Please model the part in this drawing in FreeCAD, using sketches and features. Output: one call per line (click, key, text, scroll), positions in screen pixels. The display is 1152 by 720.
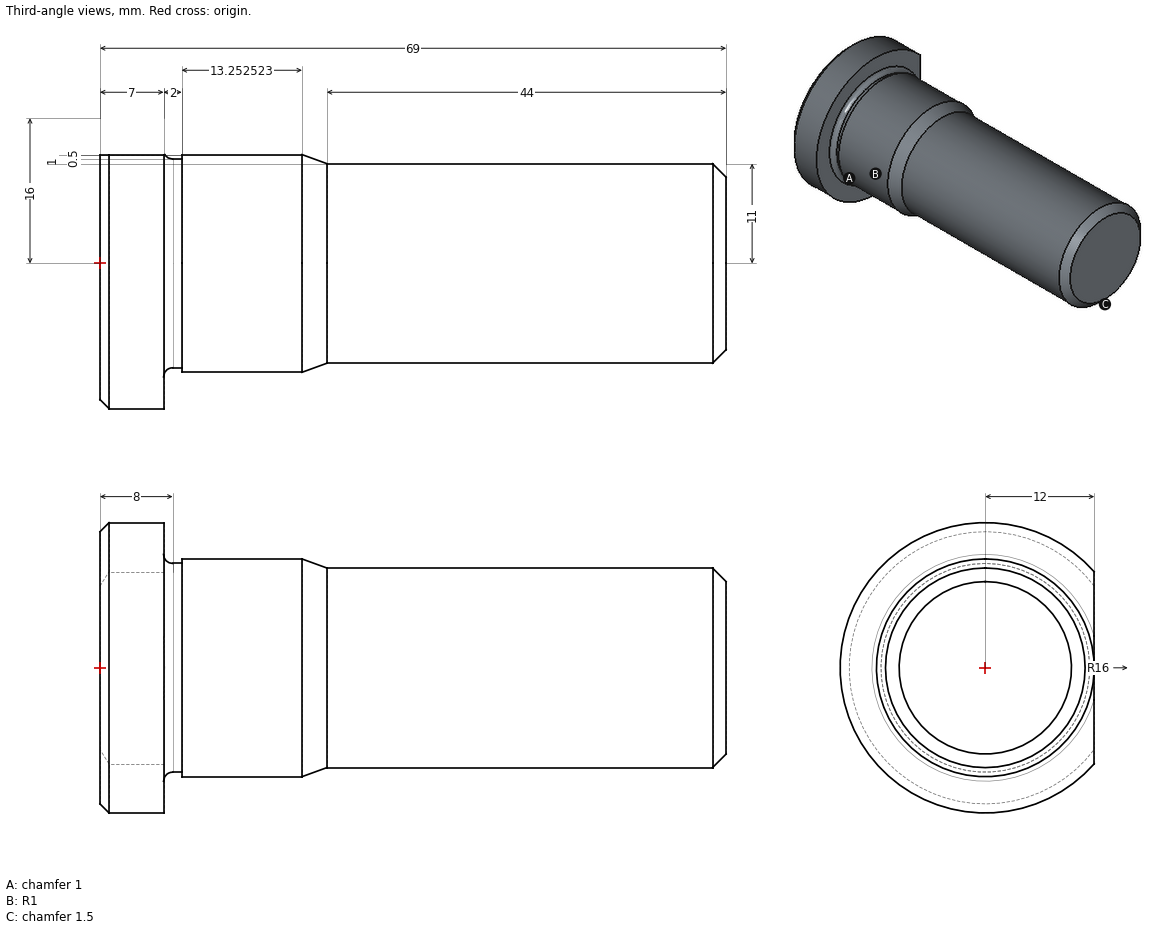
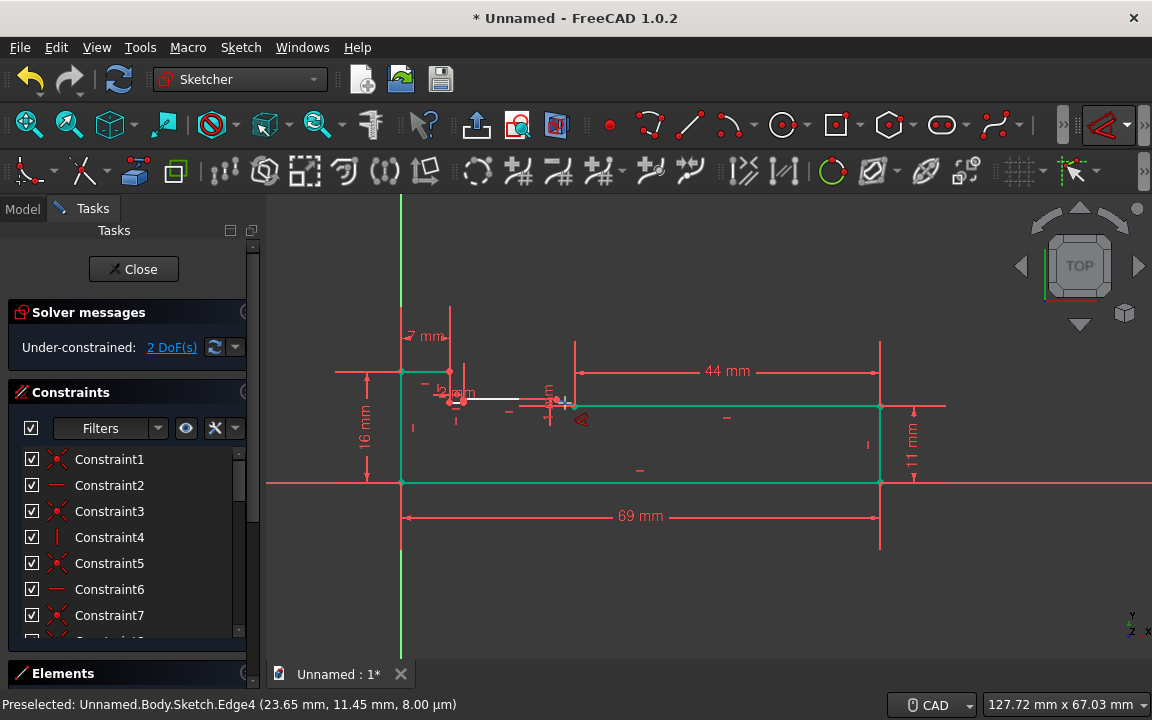
scroll(464, 401, up, 13)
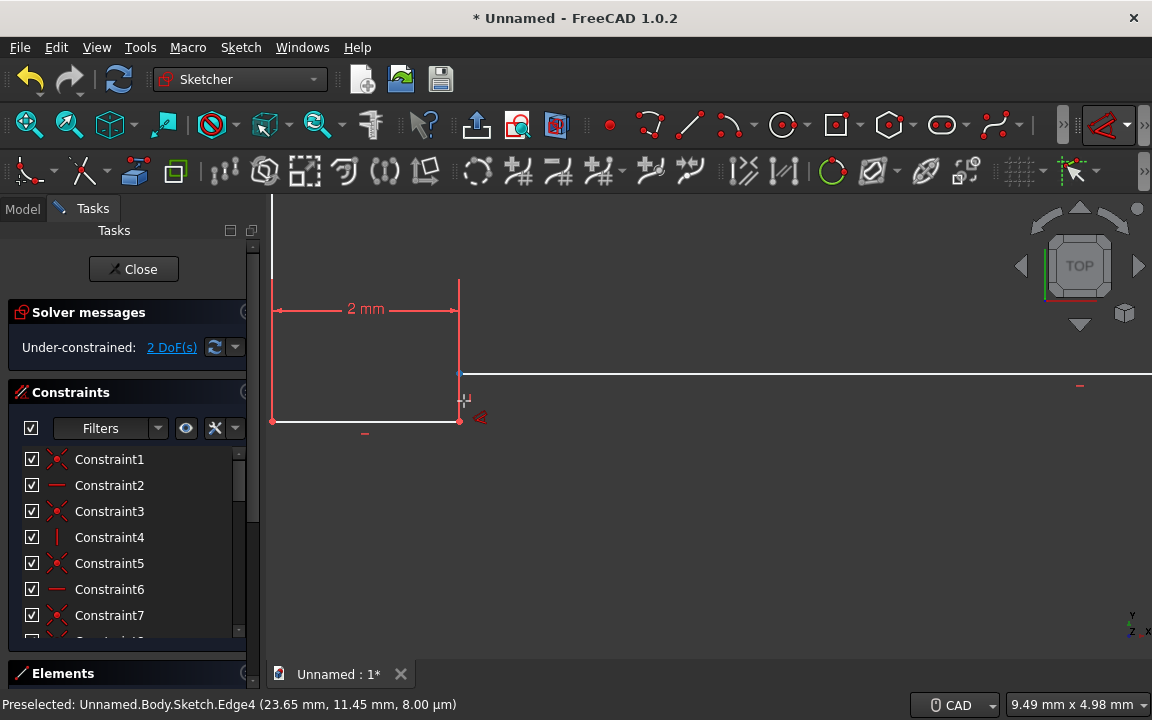
click(459, 398)
click(425, 398)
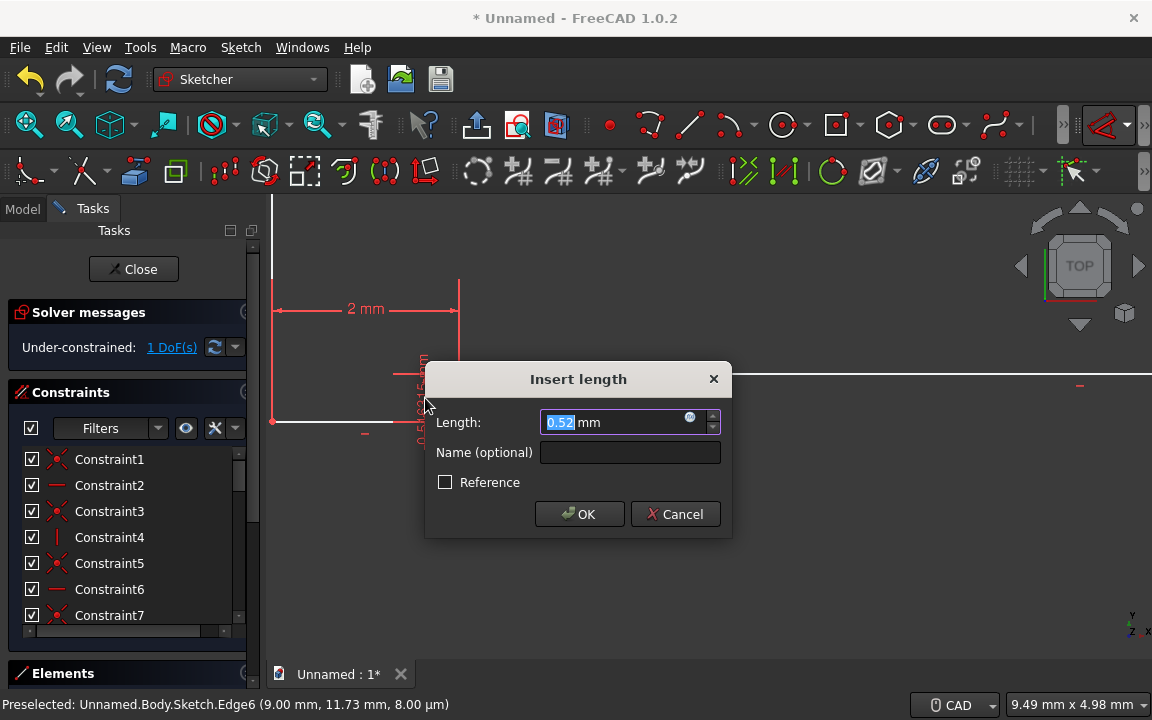
text(0.5)
key(Return)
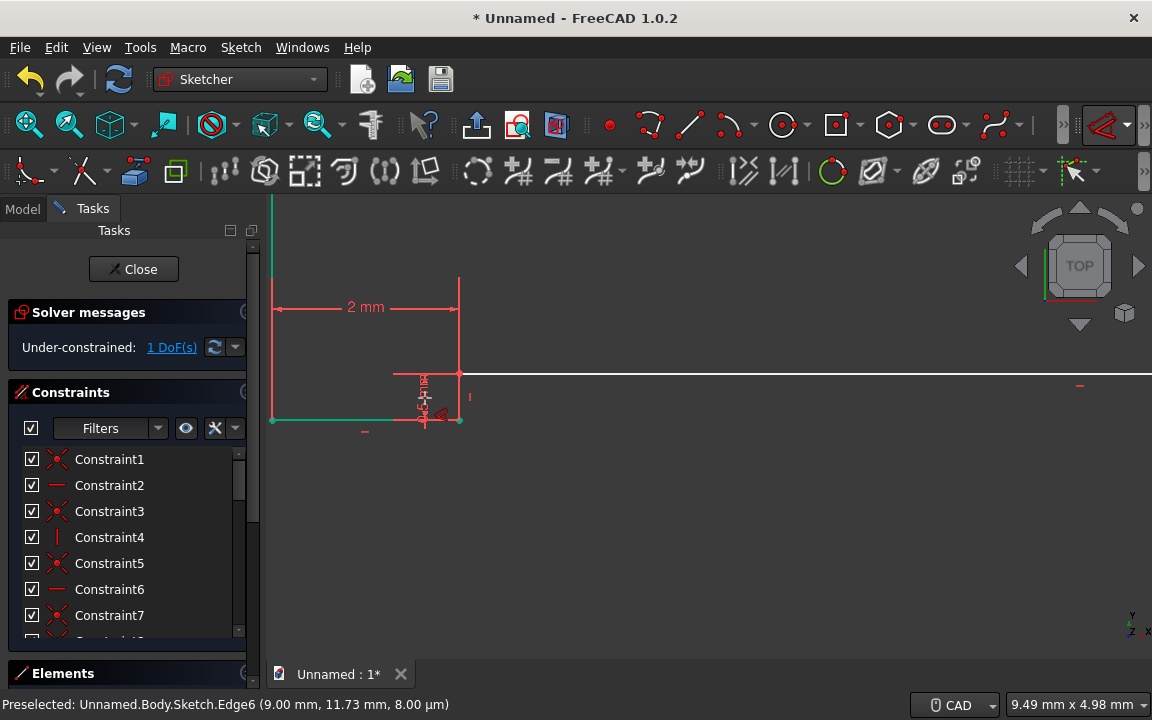
scroll(464, 401, down, 13)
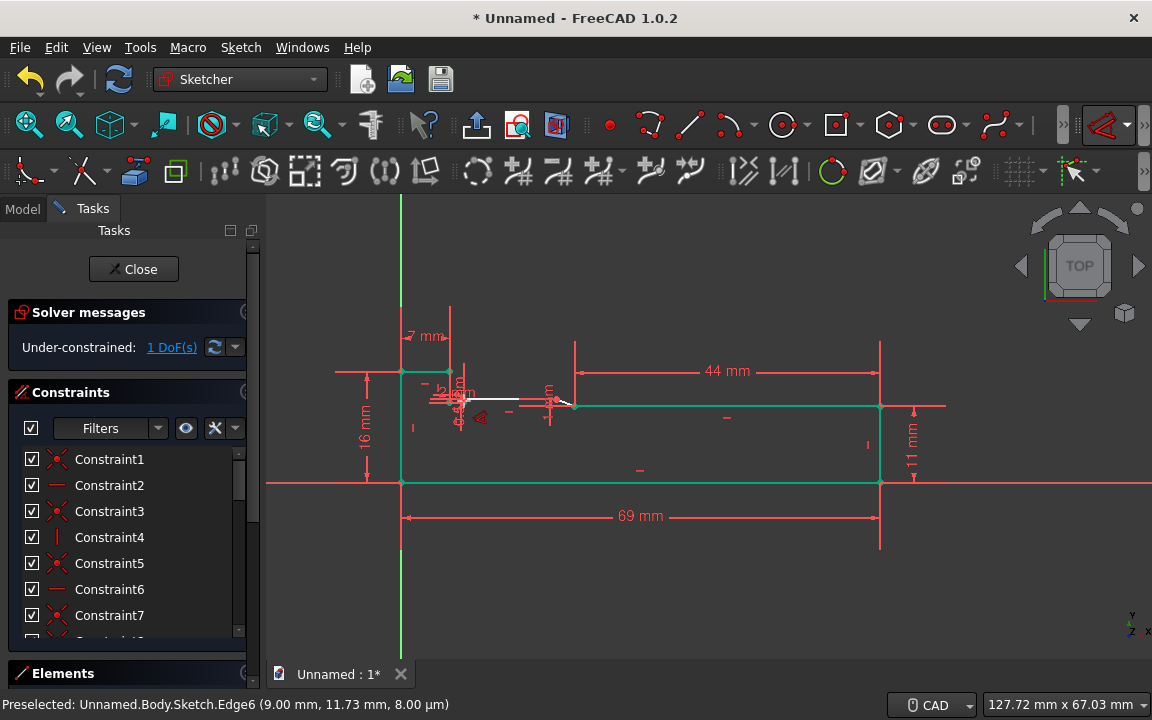
click(492, 399)
click(510, 365)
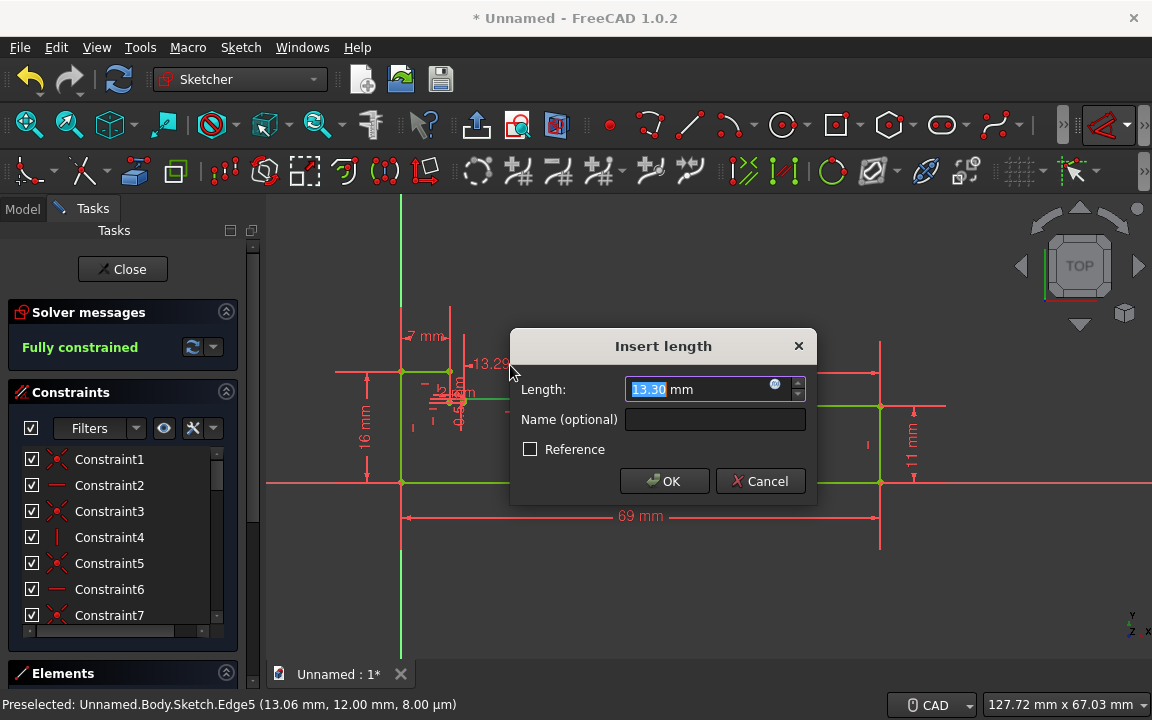
text(13.252523)
key(Return)
key(Escape)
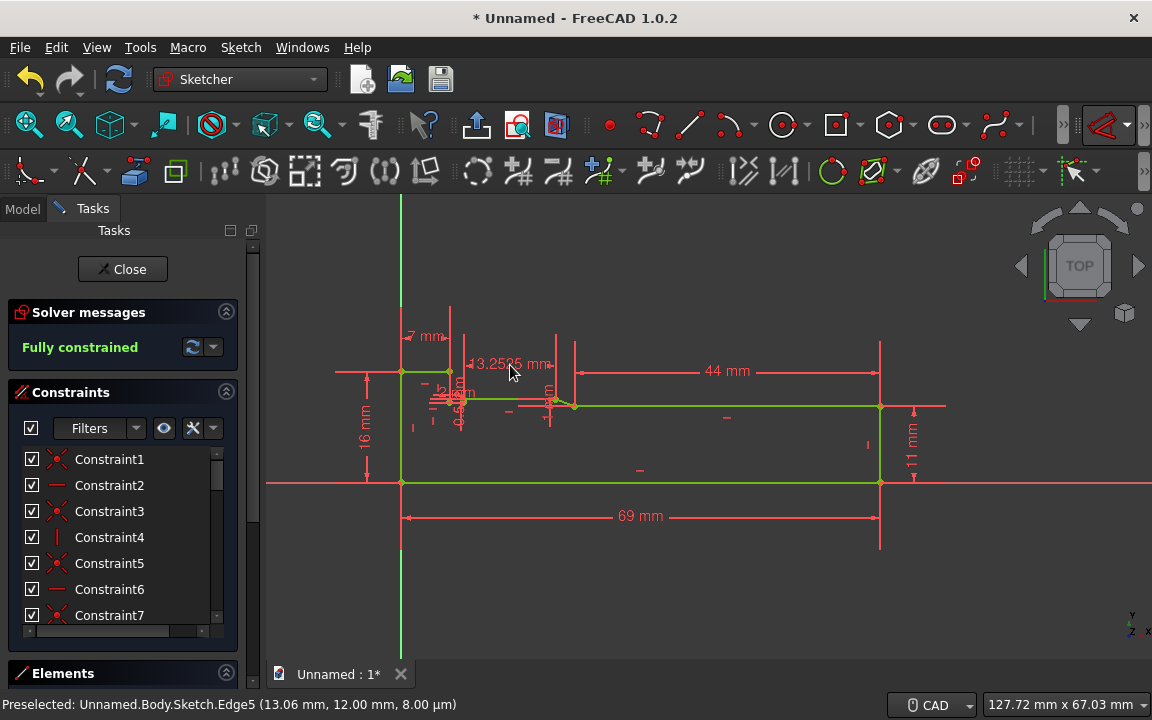
click(123, 269)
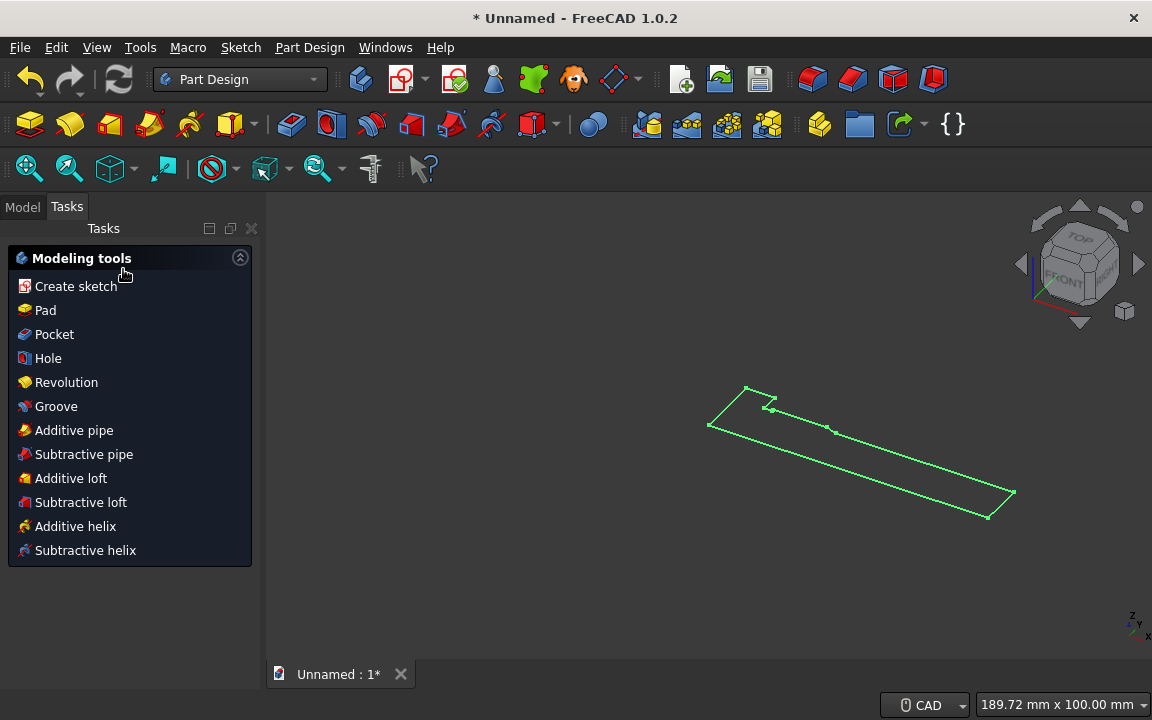
click(70, 124)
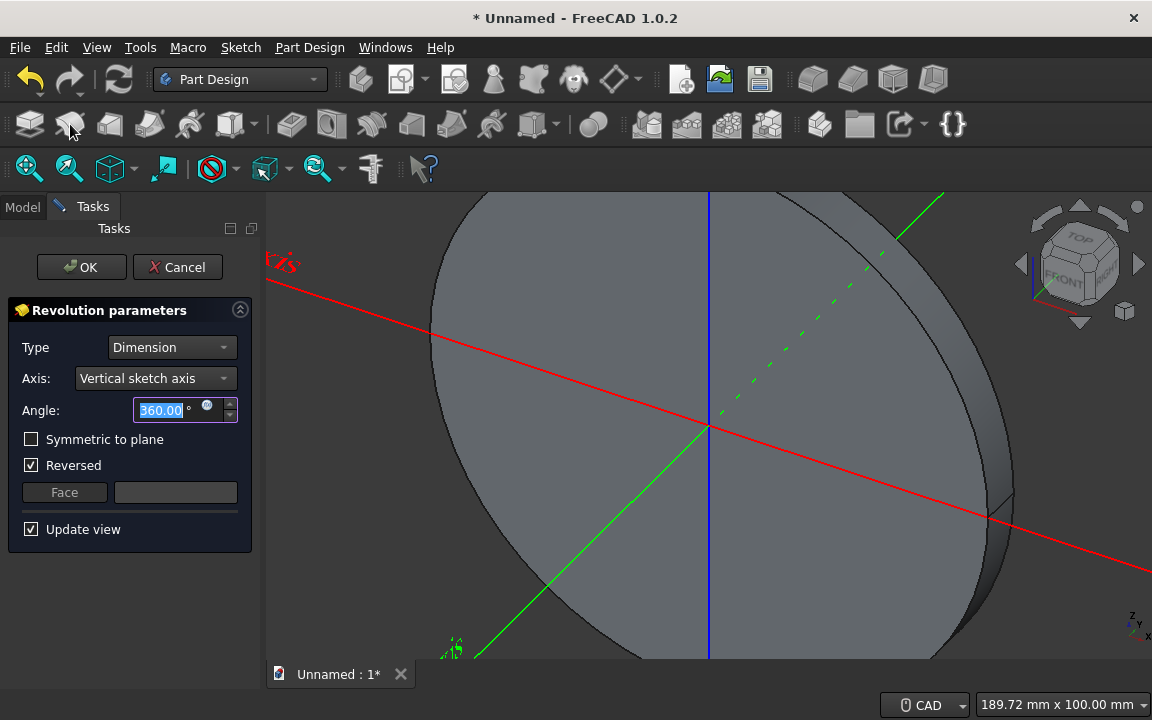
click(156, 378)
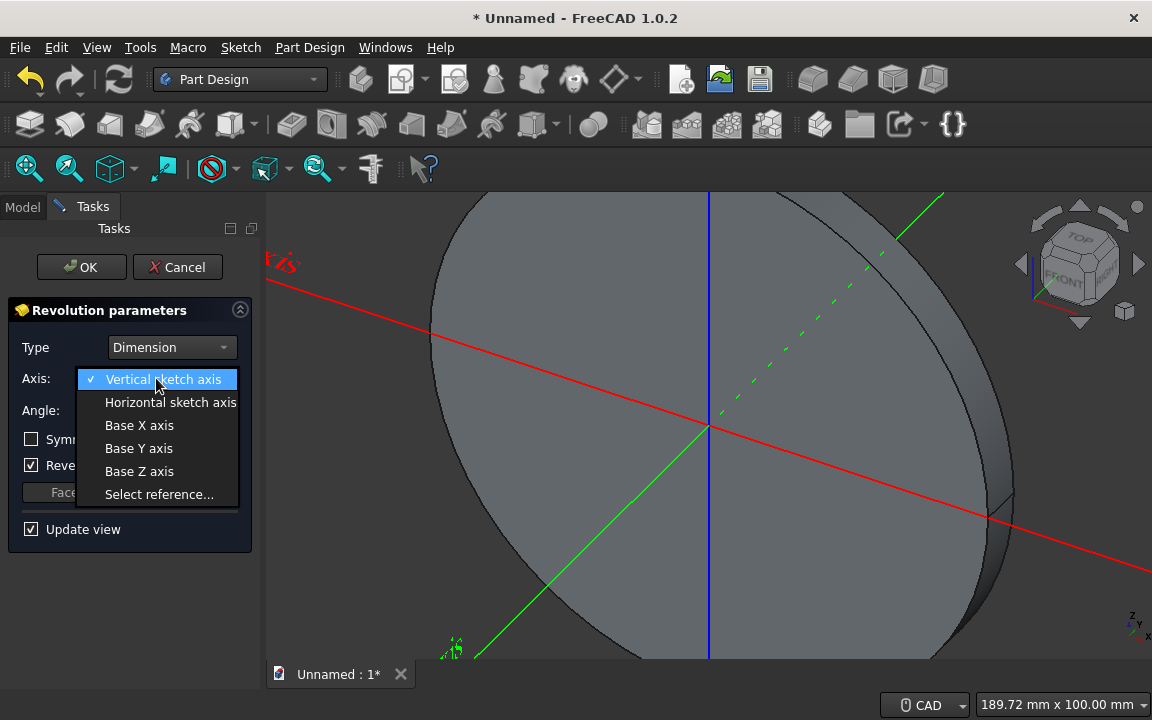
click(156, 402)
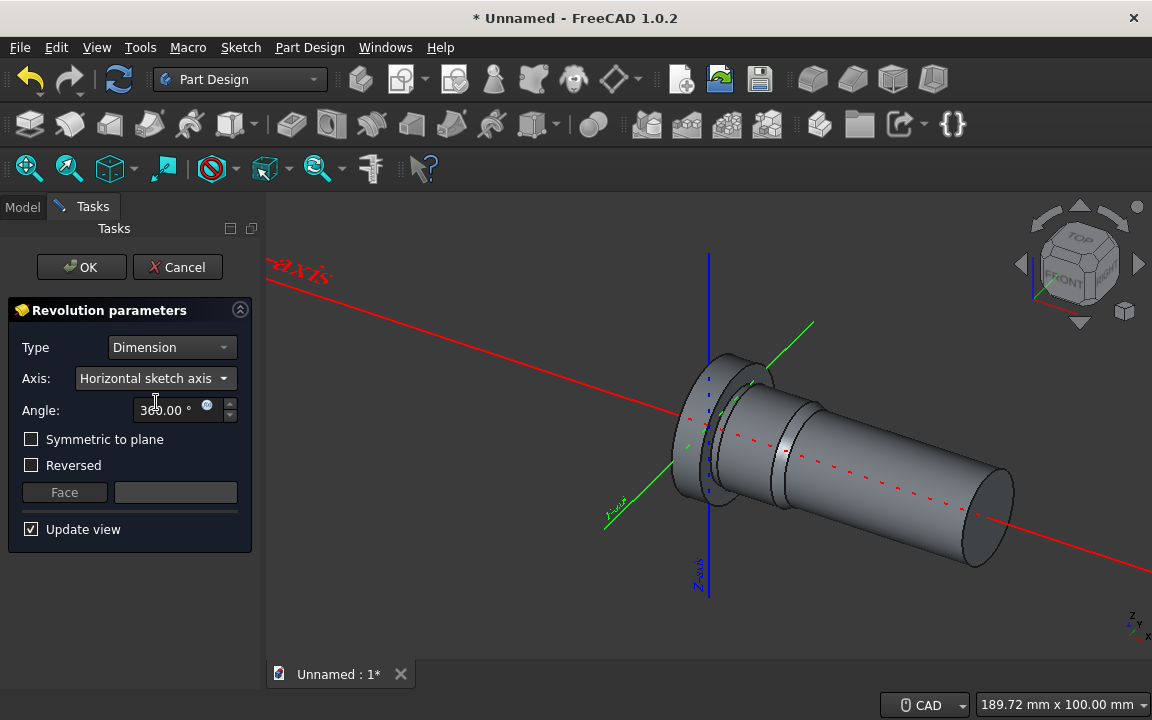
click(82, 267)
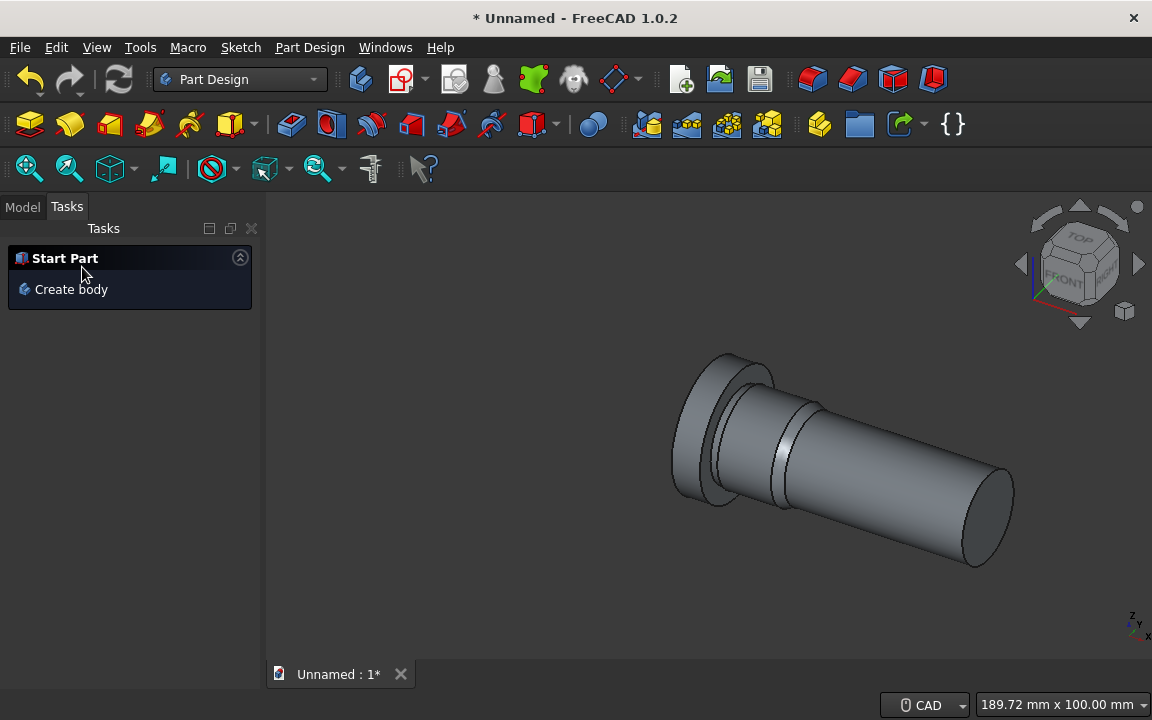
key(0)